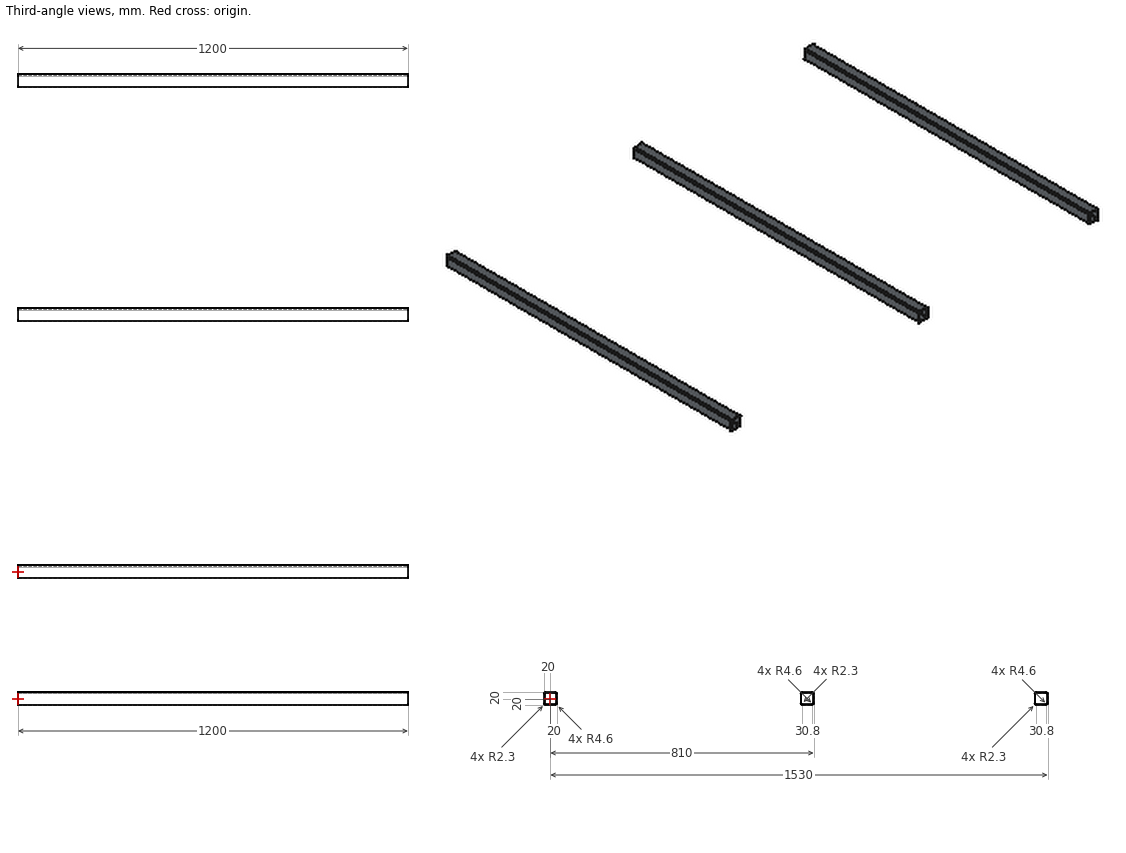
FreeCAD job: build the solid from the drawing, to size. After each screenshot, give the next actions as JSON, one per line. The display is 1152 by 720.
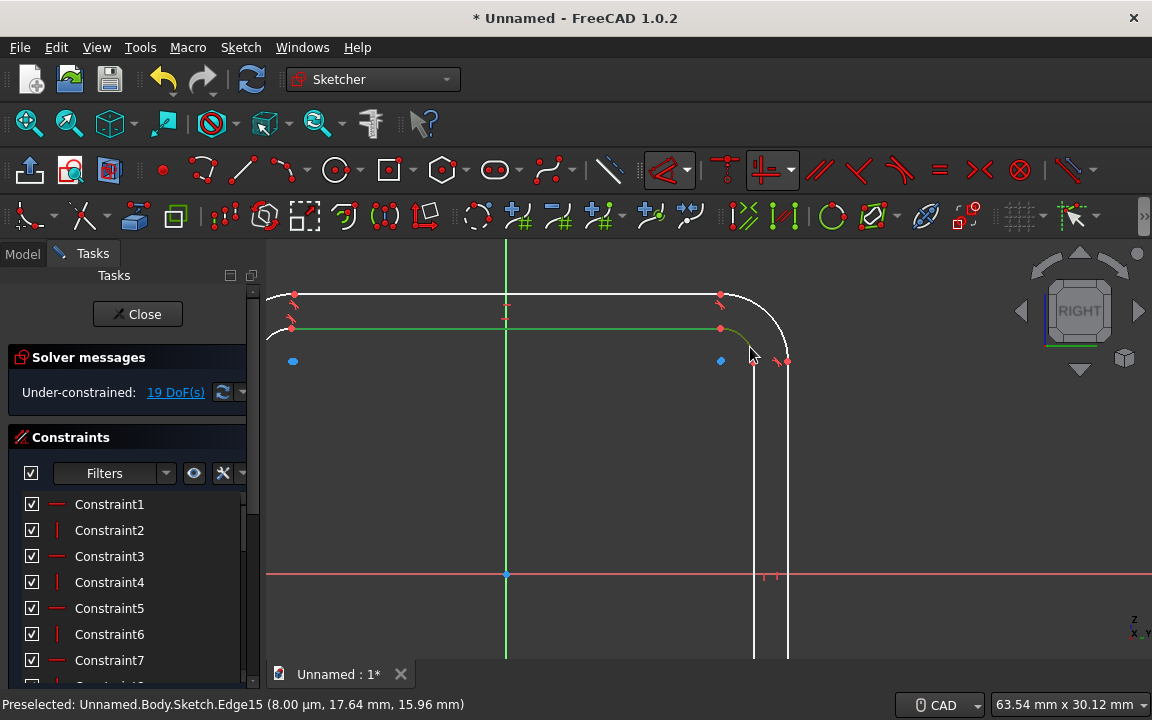
{"action": "key", "text": "t"}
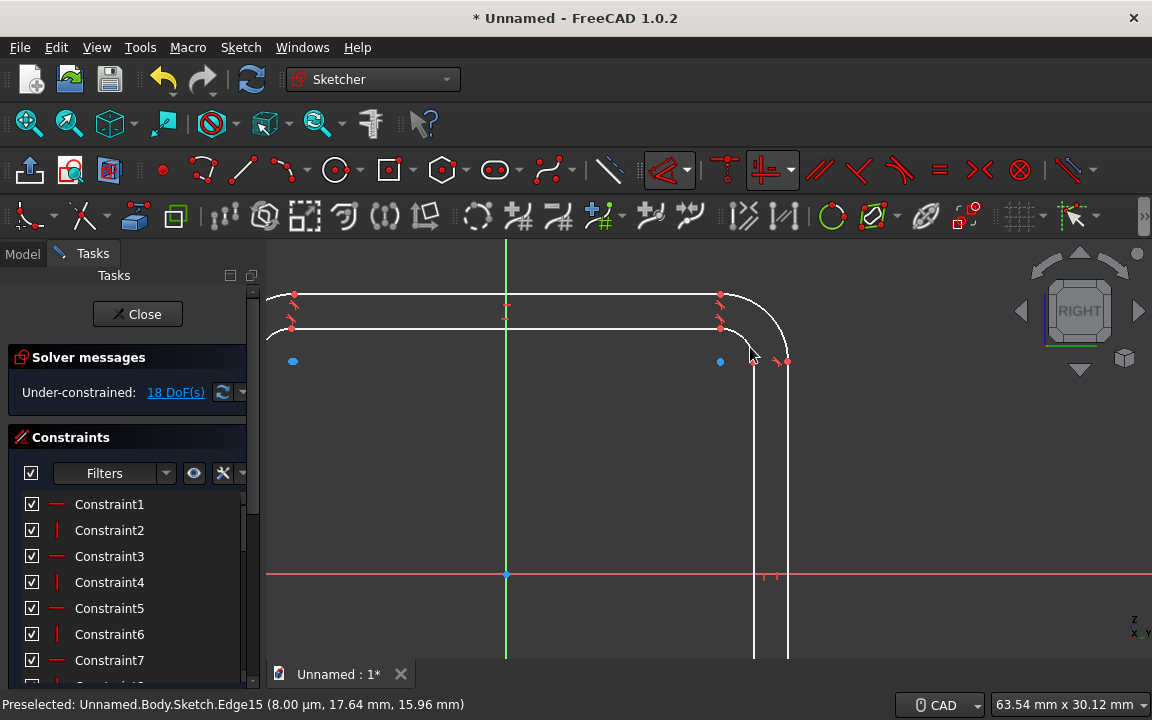
{"action": "left_click", "coordinate": [754, 491]}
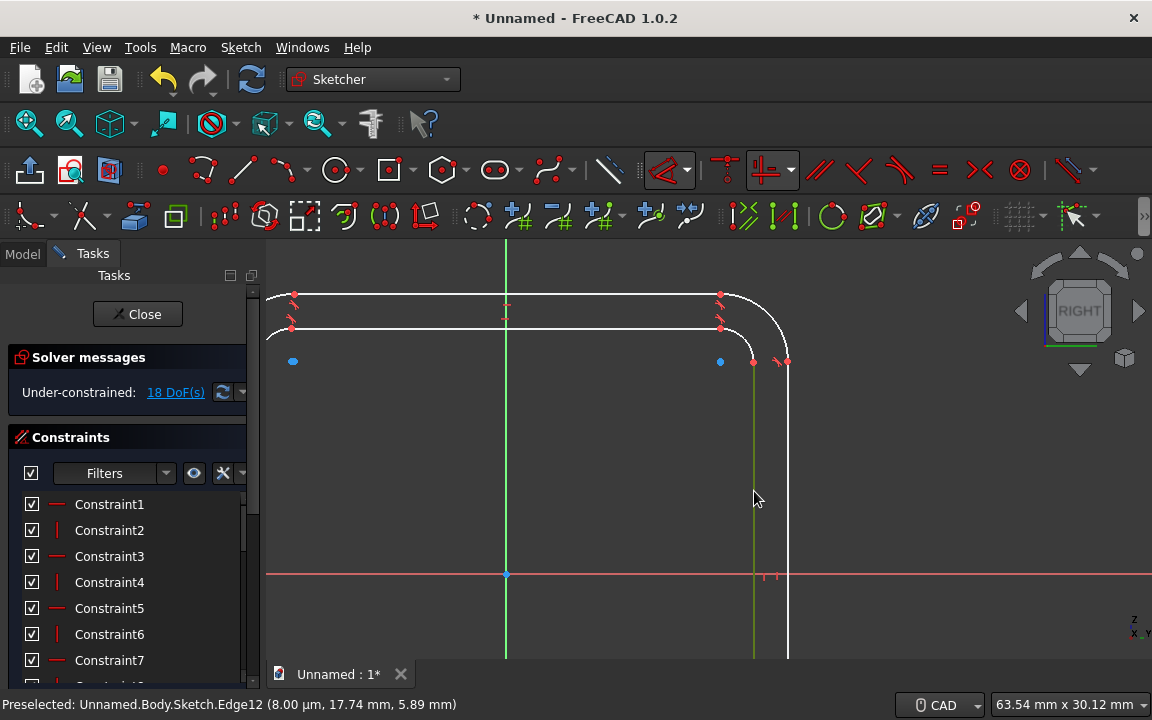
{"action": "left_click", "coordinate": [750, 347]}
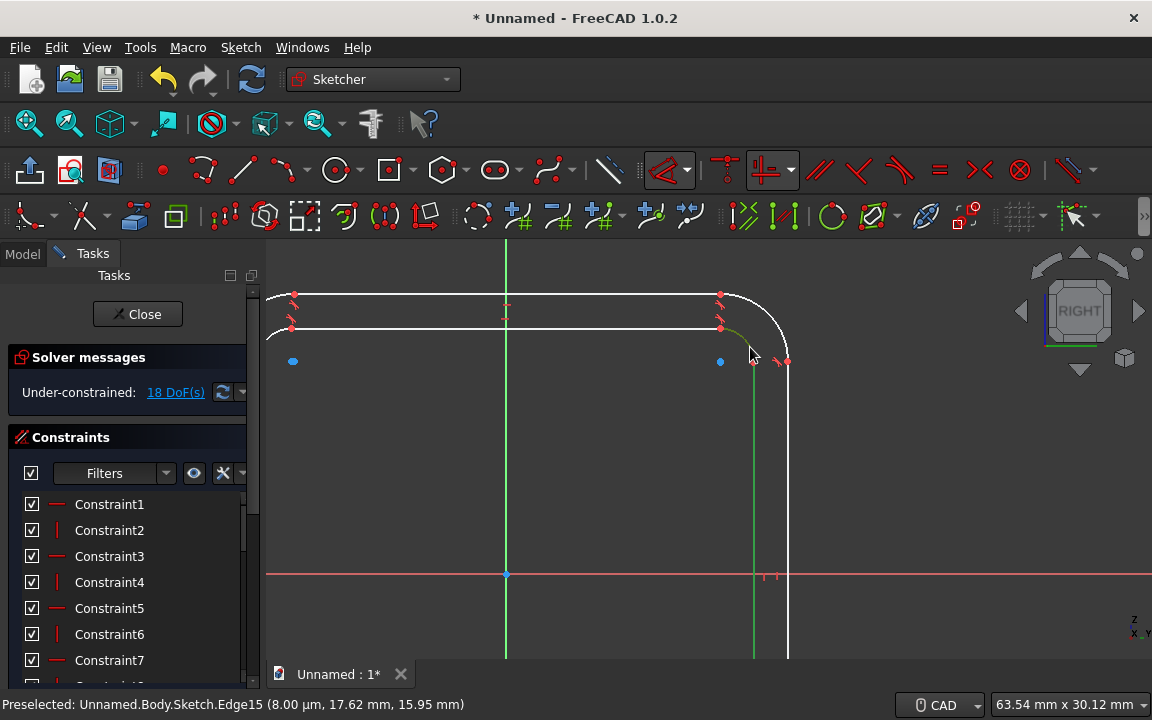
{"action": "key", "text": "t"}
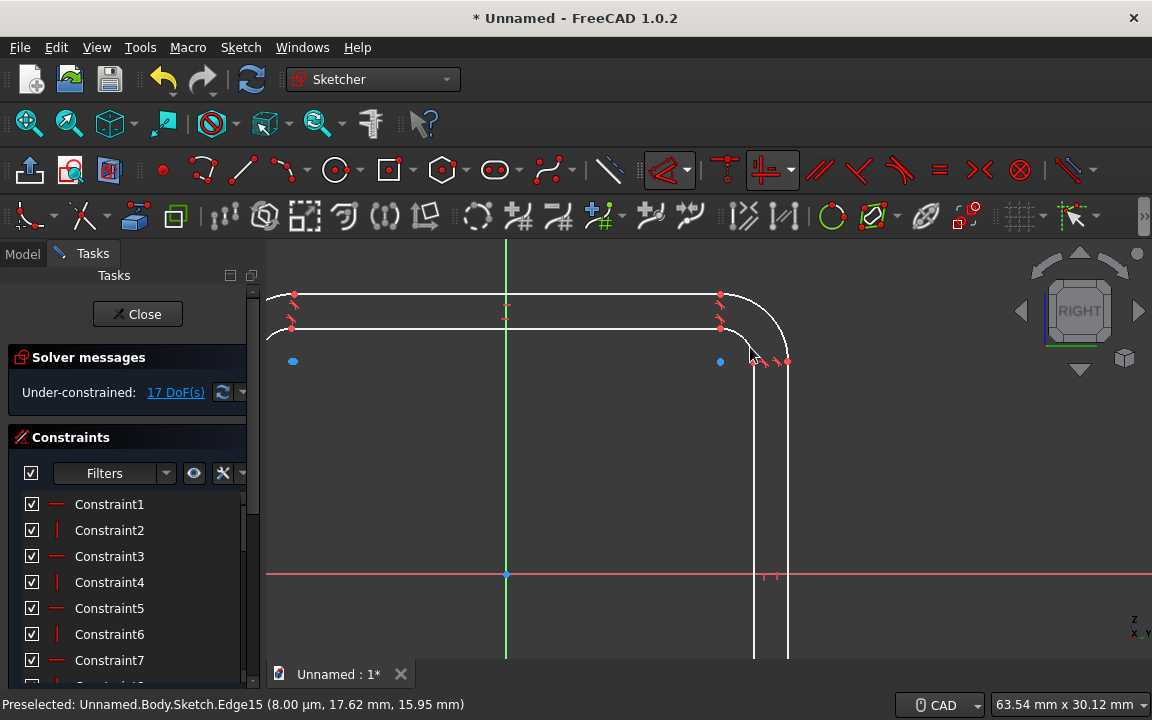
{"action": "left_click", "coordinate": [754, 491]}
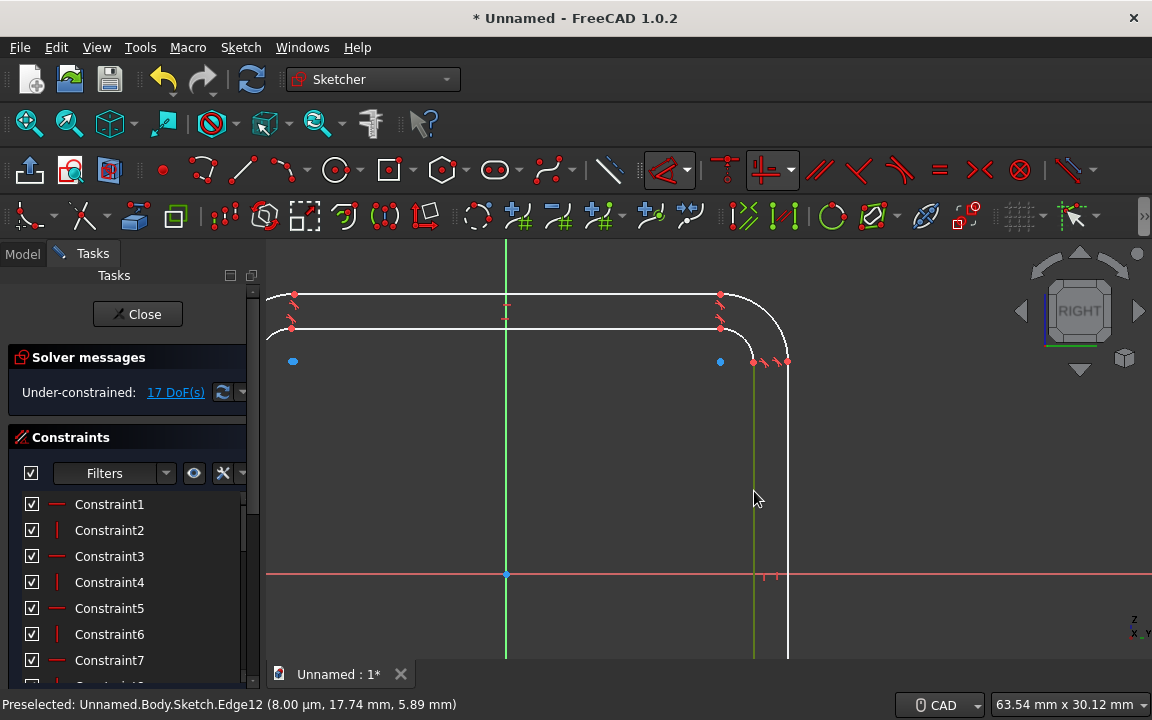
{"action": "scroll", "coordinate": [750, 347], "scroll_direction": "down", "scroll_amount": 4}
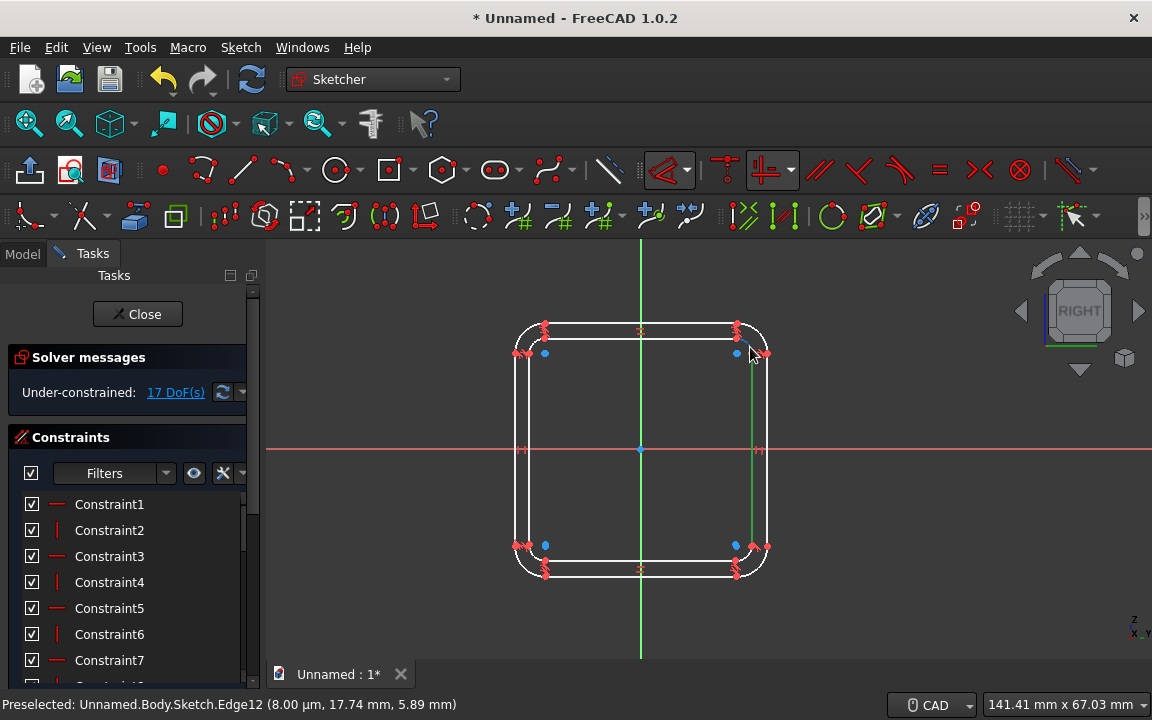
{"action": "scroll", "coordinate": [743, 559], "scroll_direction": "up", "scroll_amount": 4}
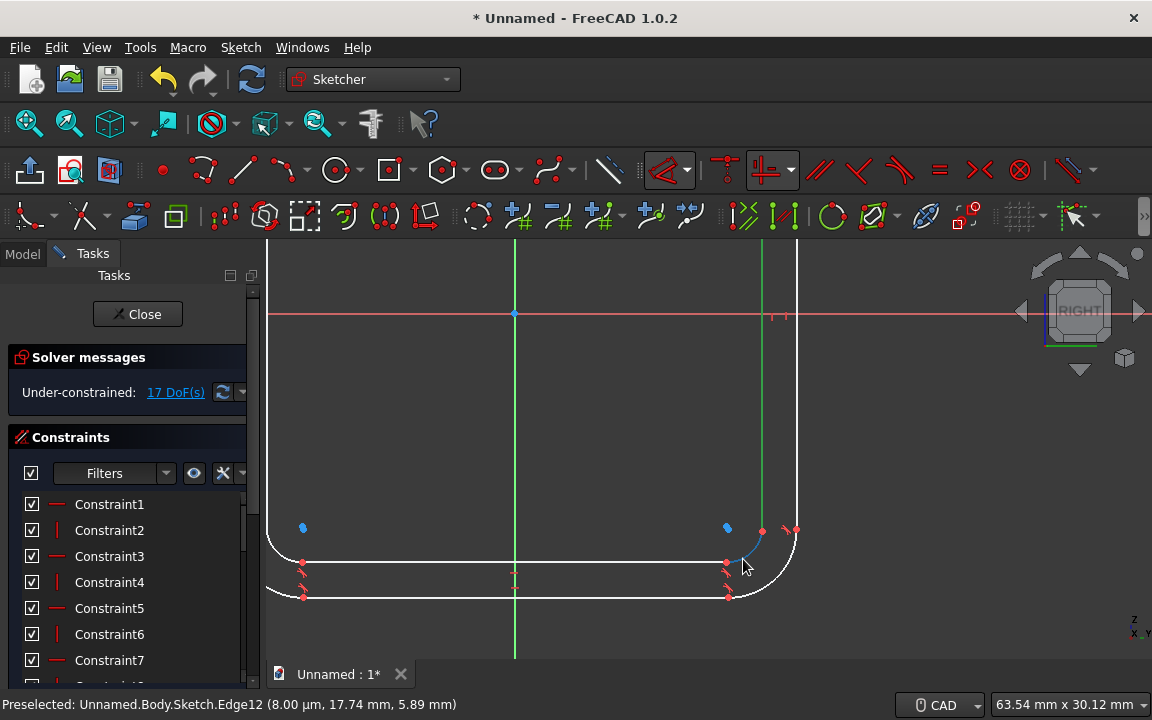
{"action": "left_click", "coordinate": [742, 559]}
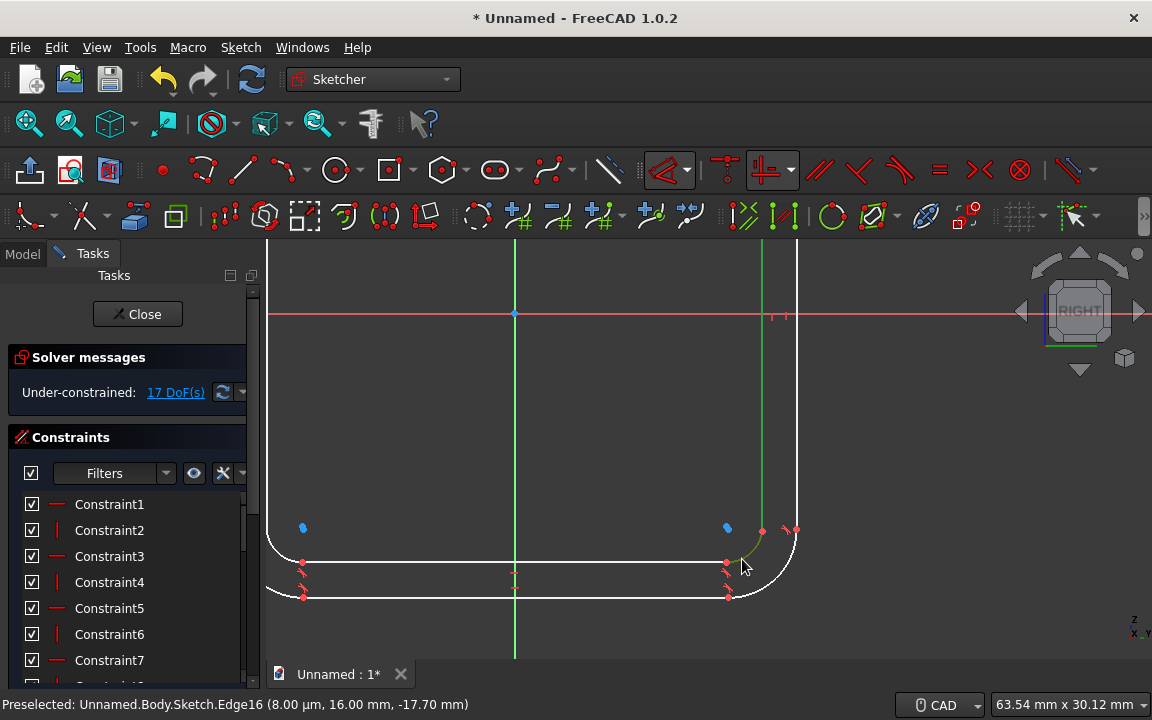
{"action": "left_click", "coordinate": [900, 170]}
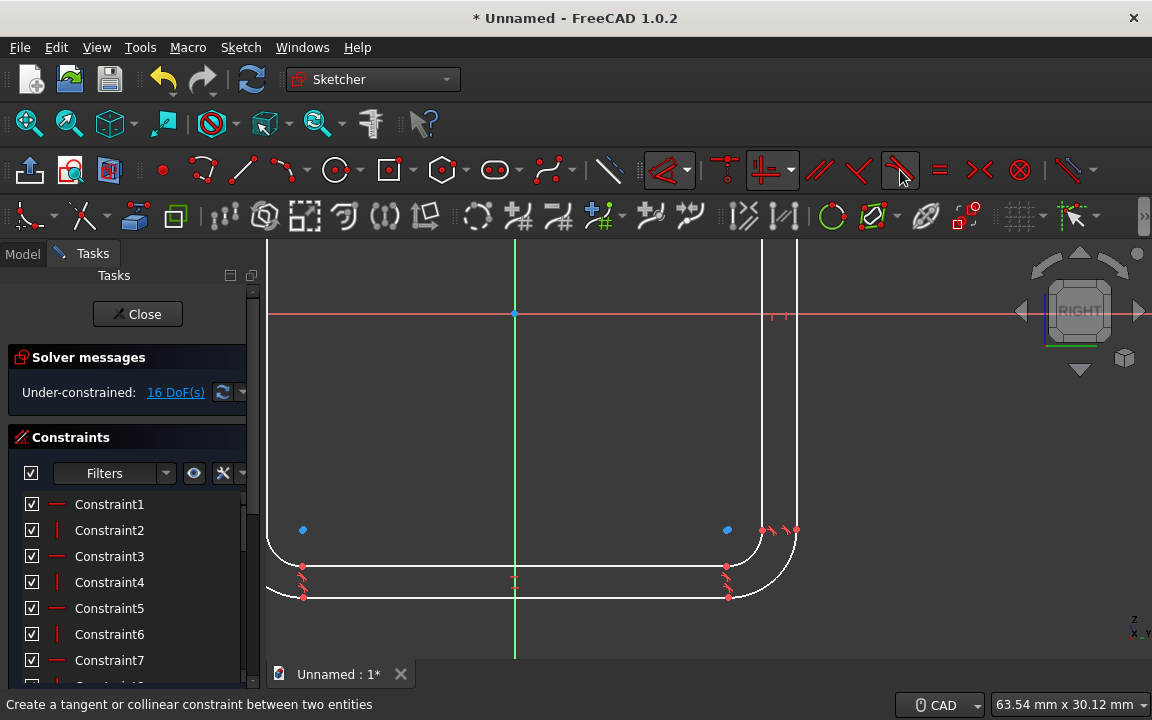
{"action": "scroll", "coordinate": [743, 559], "scroll_direction": "down", "scroll_amount": 4}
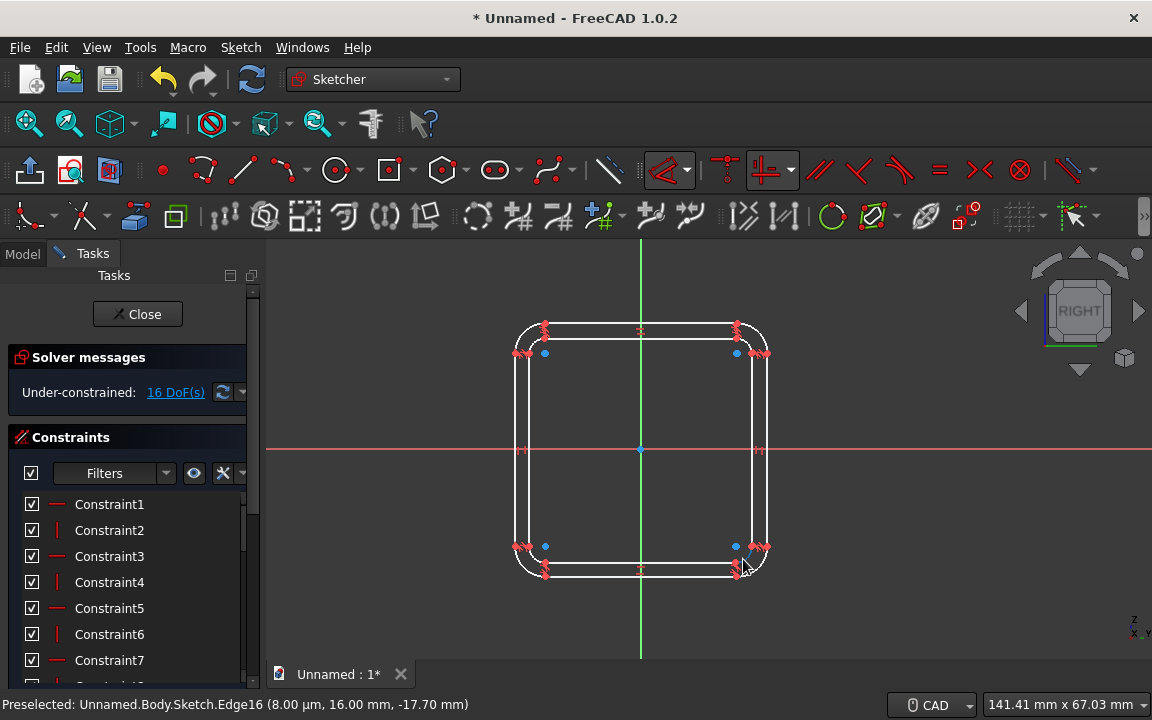
{"action": "left_click", "coordinate": [519, 560]}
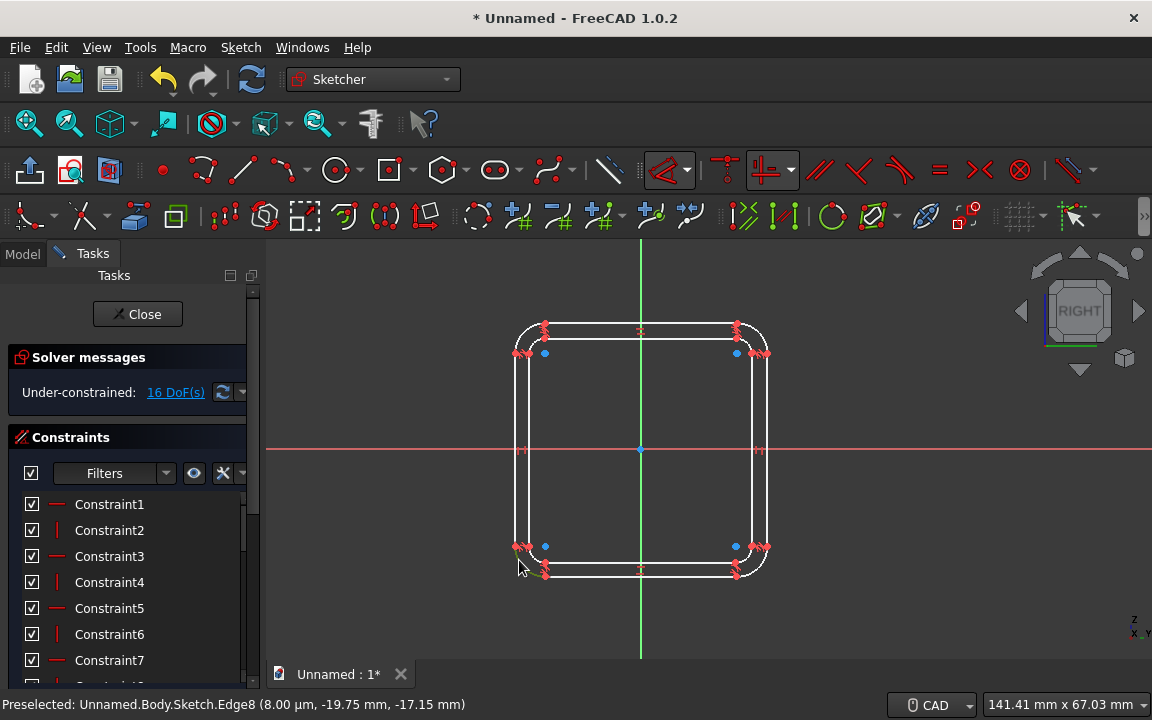
{"action": "left_click", "coordinate": [534, 558]}